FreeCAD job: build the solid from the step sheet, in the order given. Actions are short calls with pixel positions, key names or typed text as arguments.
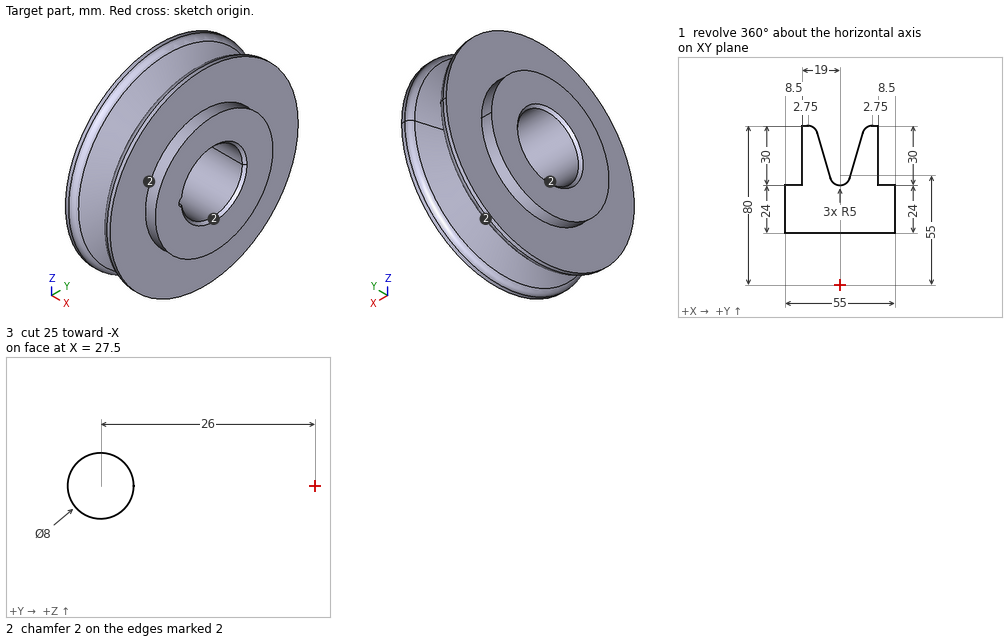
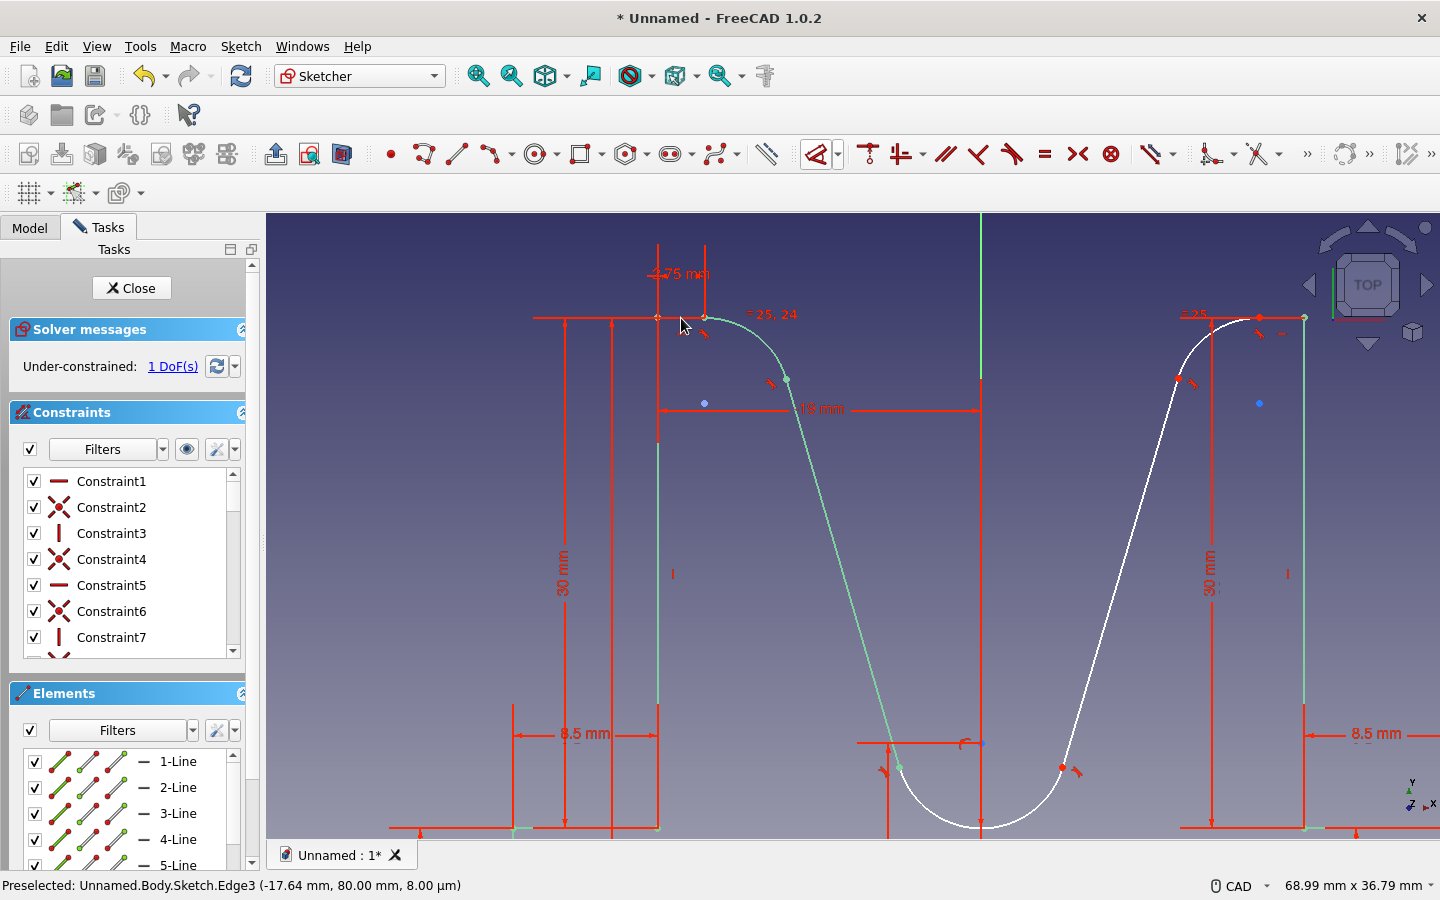
click(1273, 318)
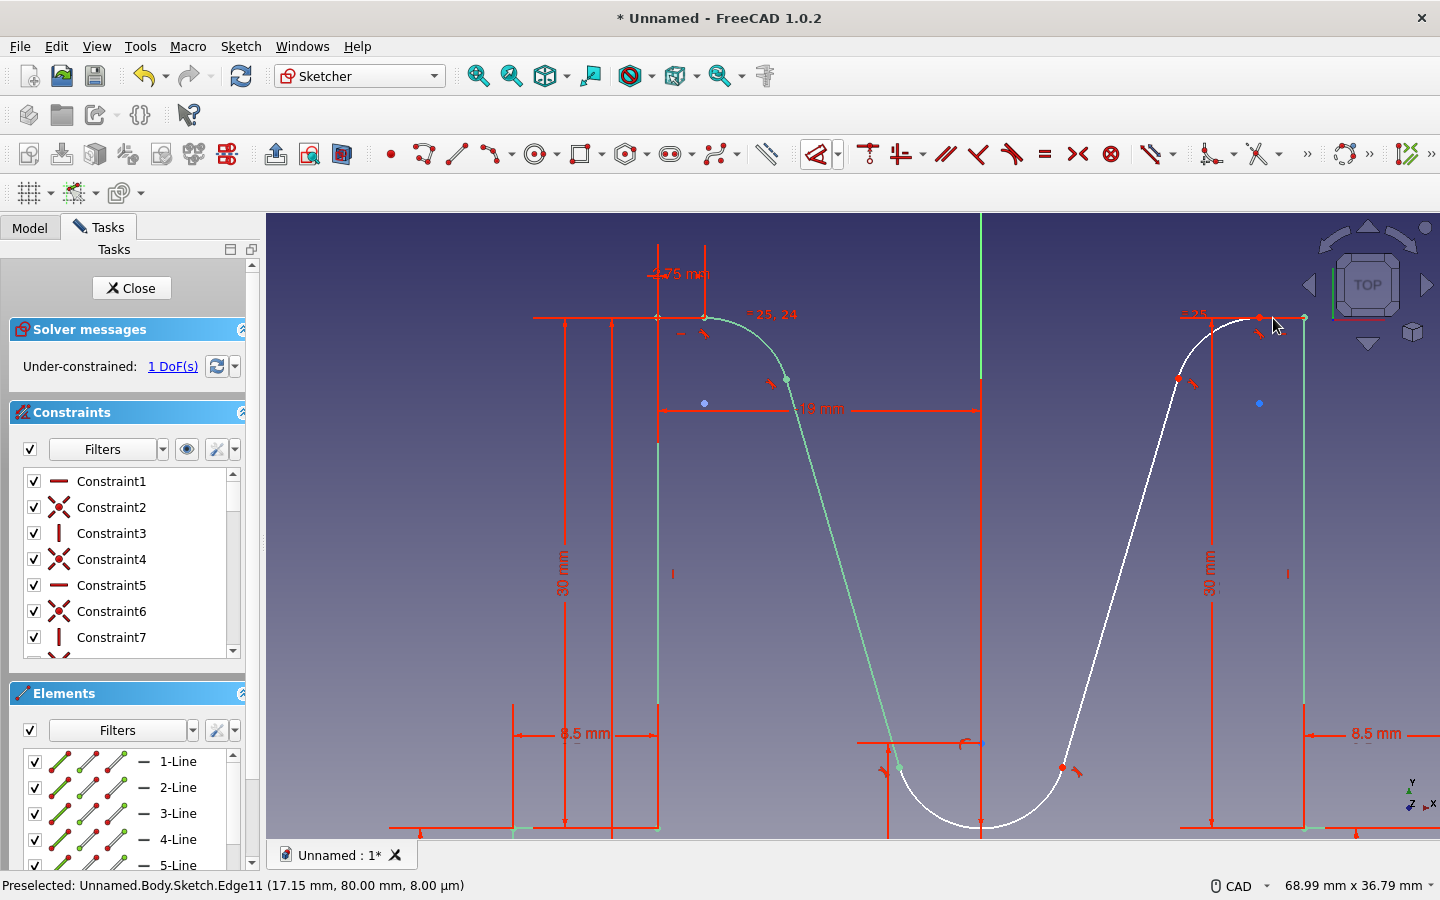
key(l)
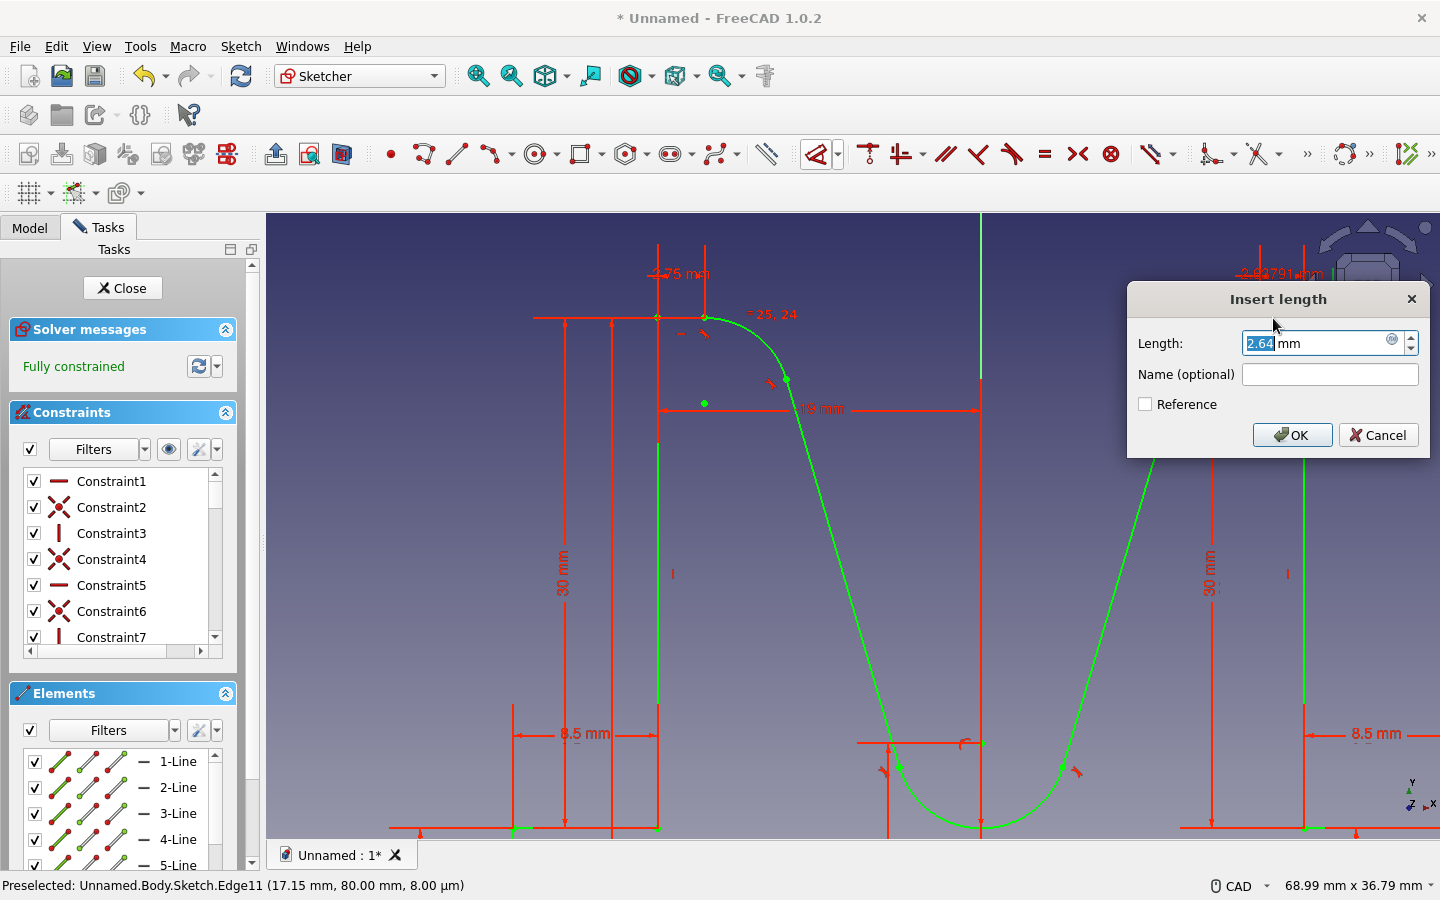
text(2.75)
key(Return)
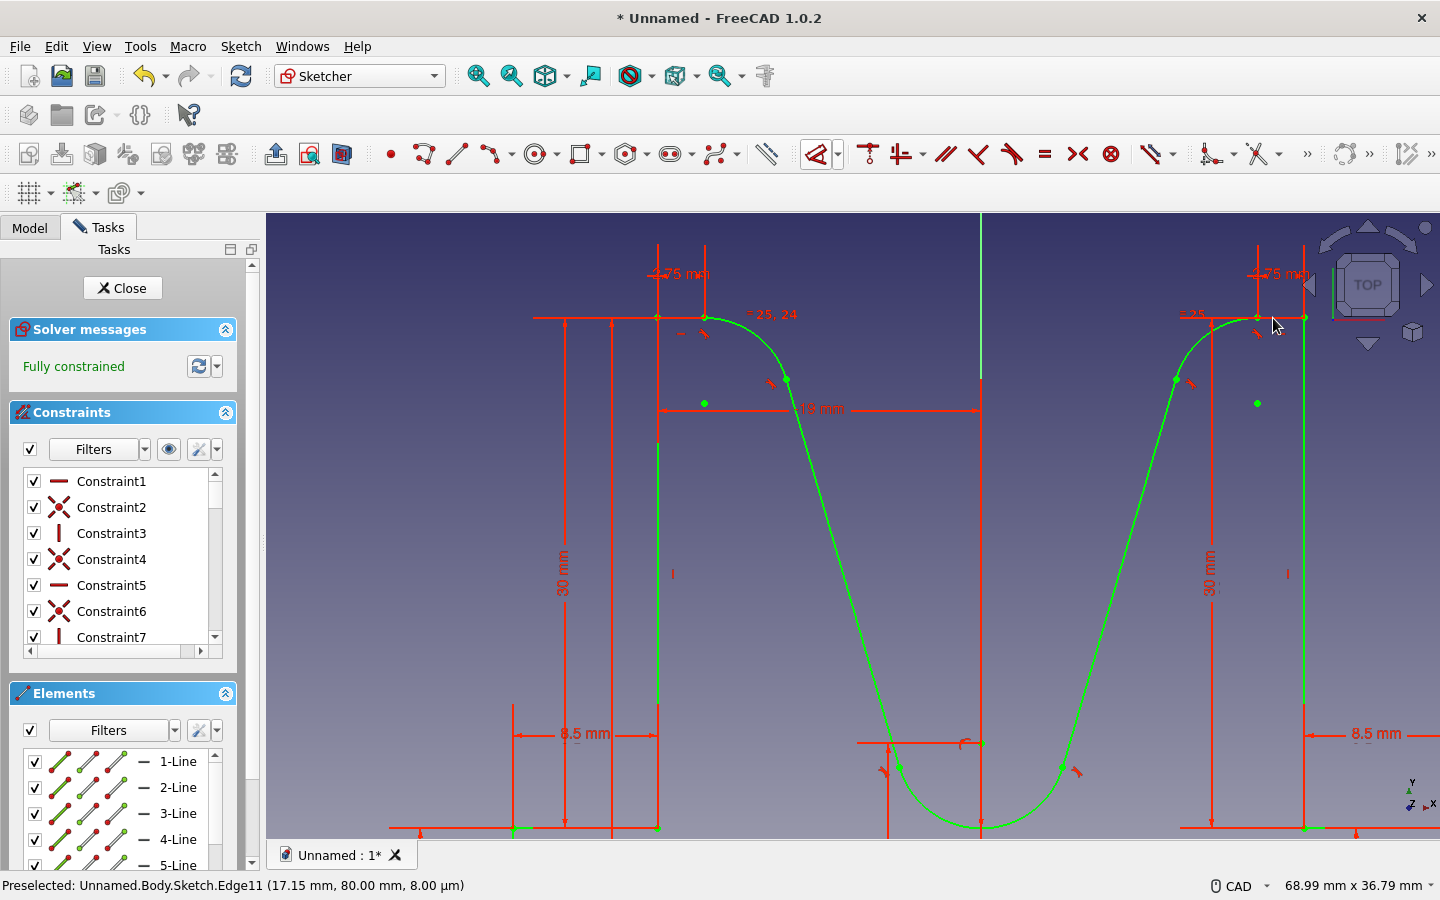
click(123, 288)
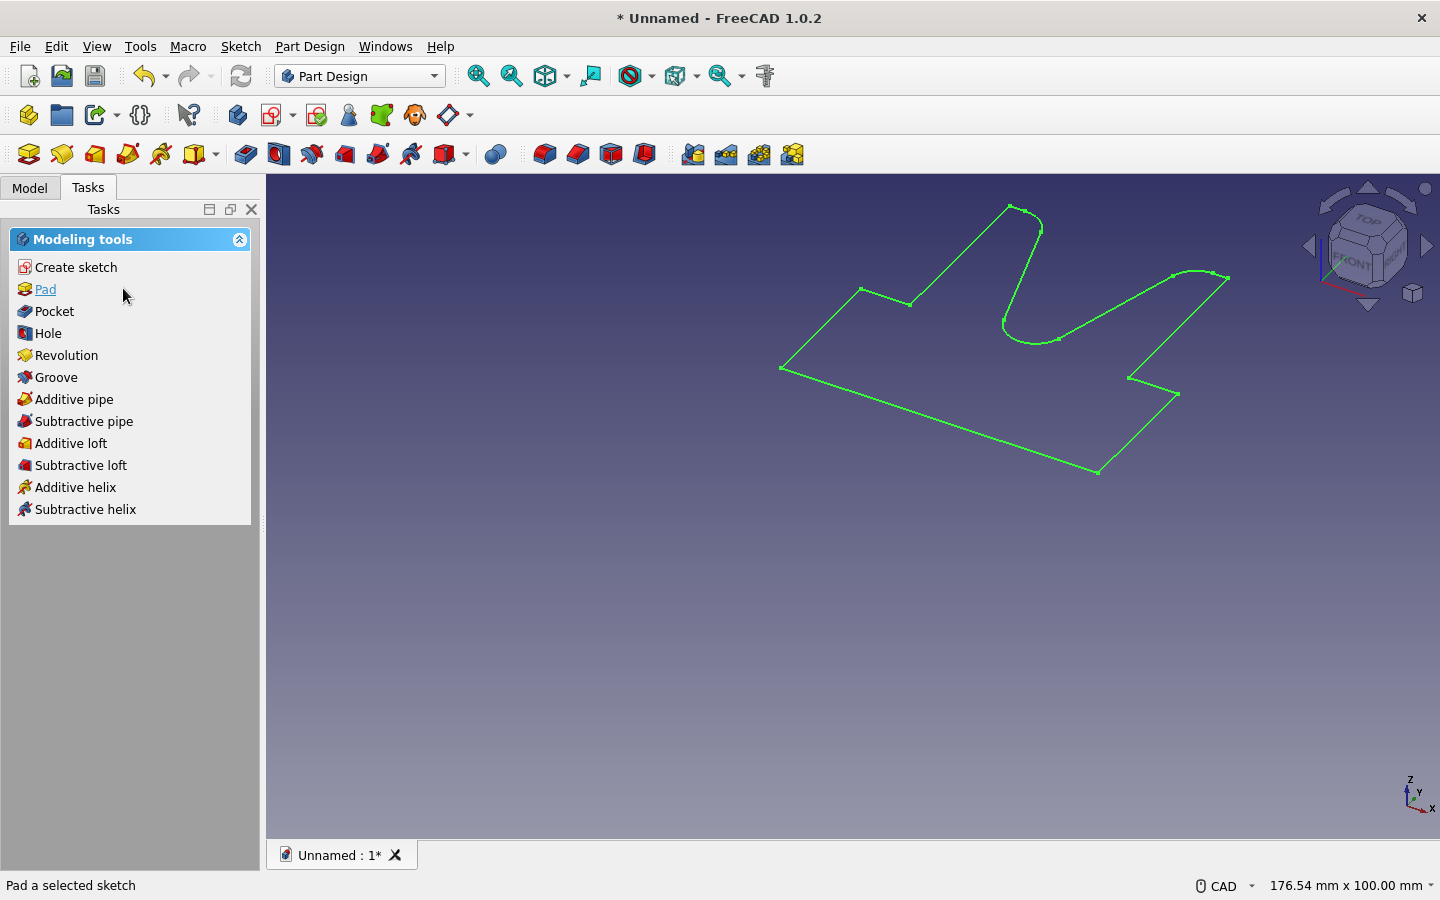
click(62, 154)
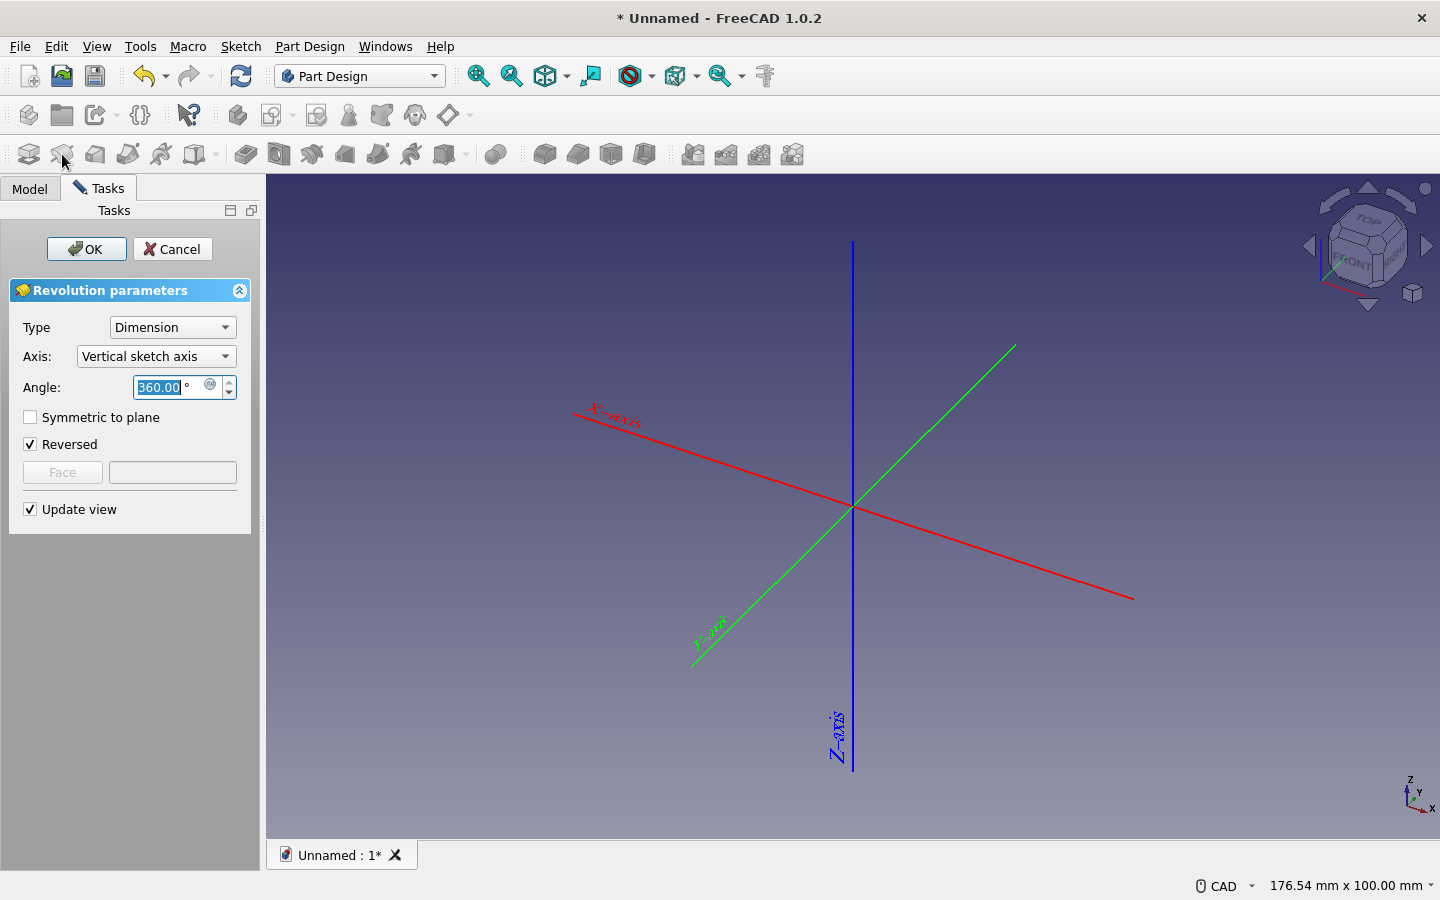
click(157, 356)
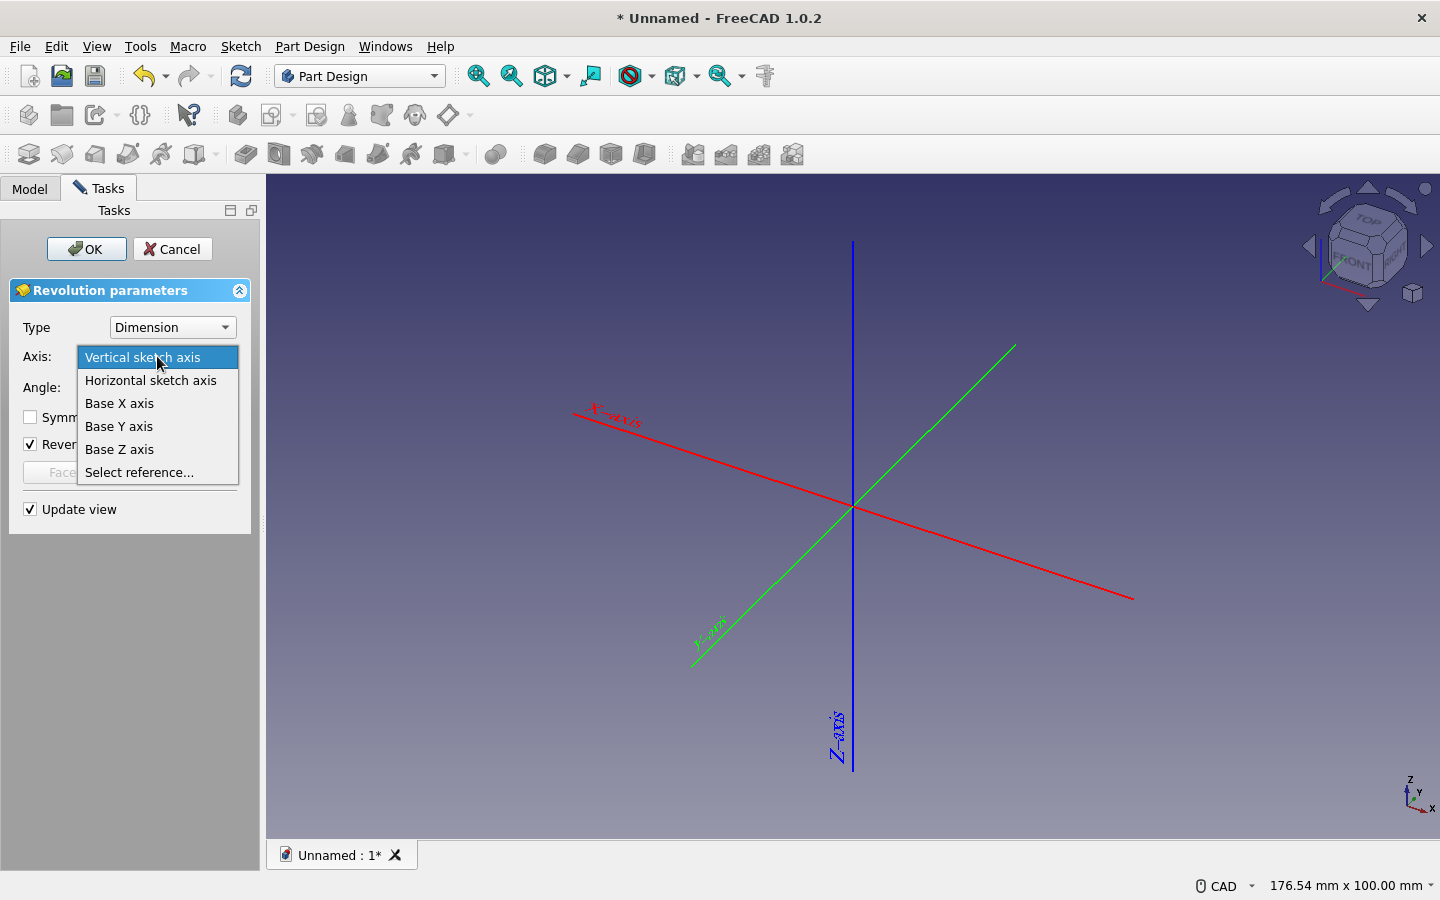
click(156, 380)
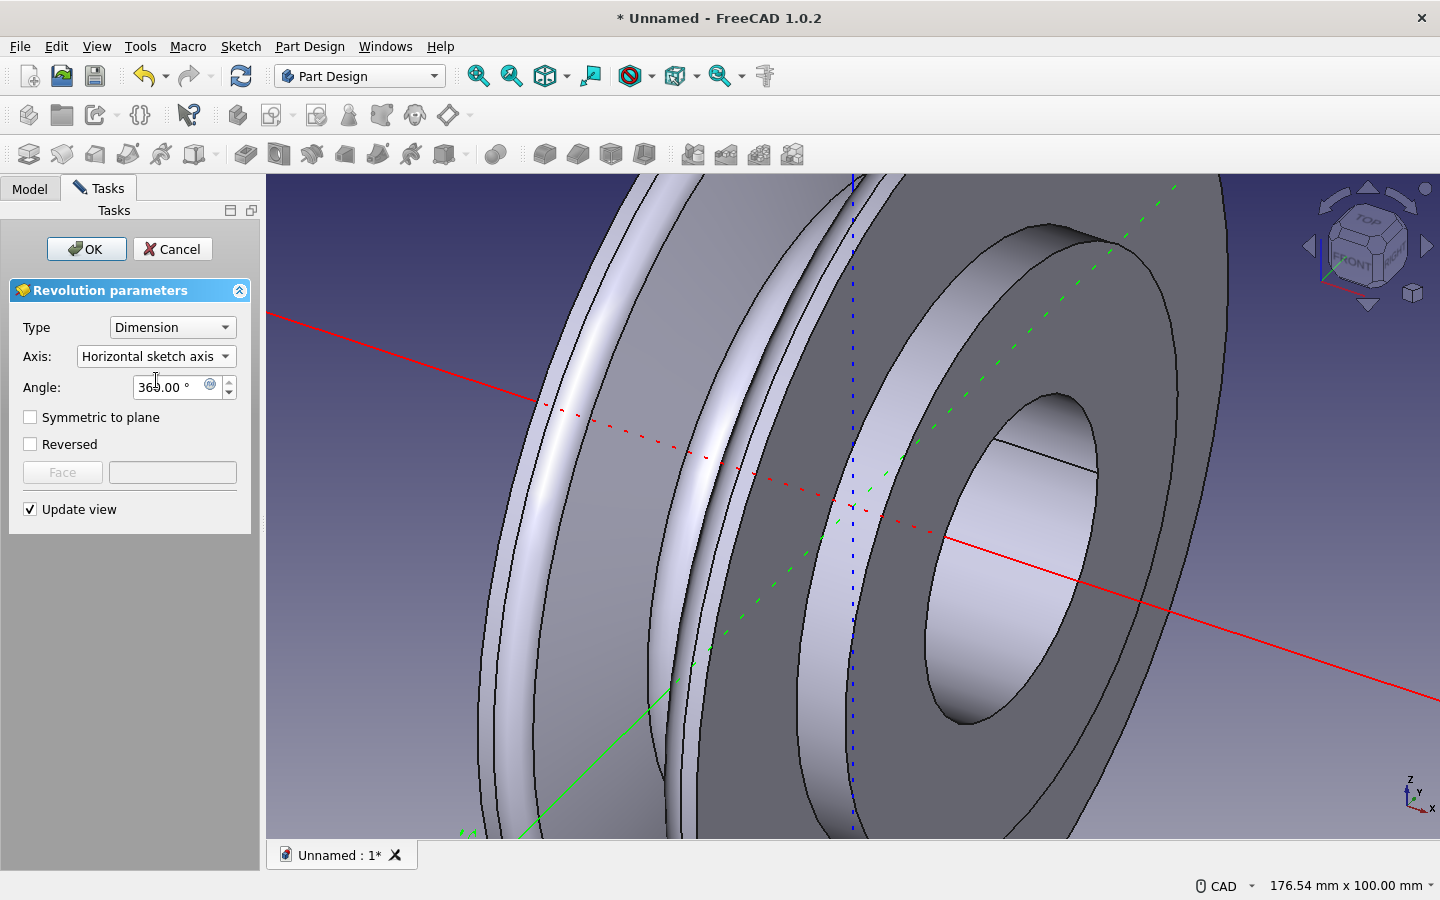
click(87, 249)